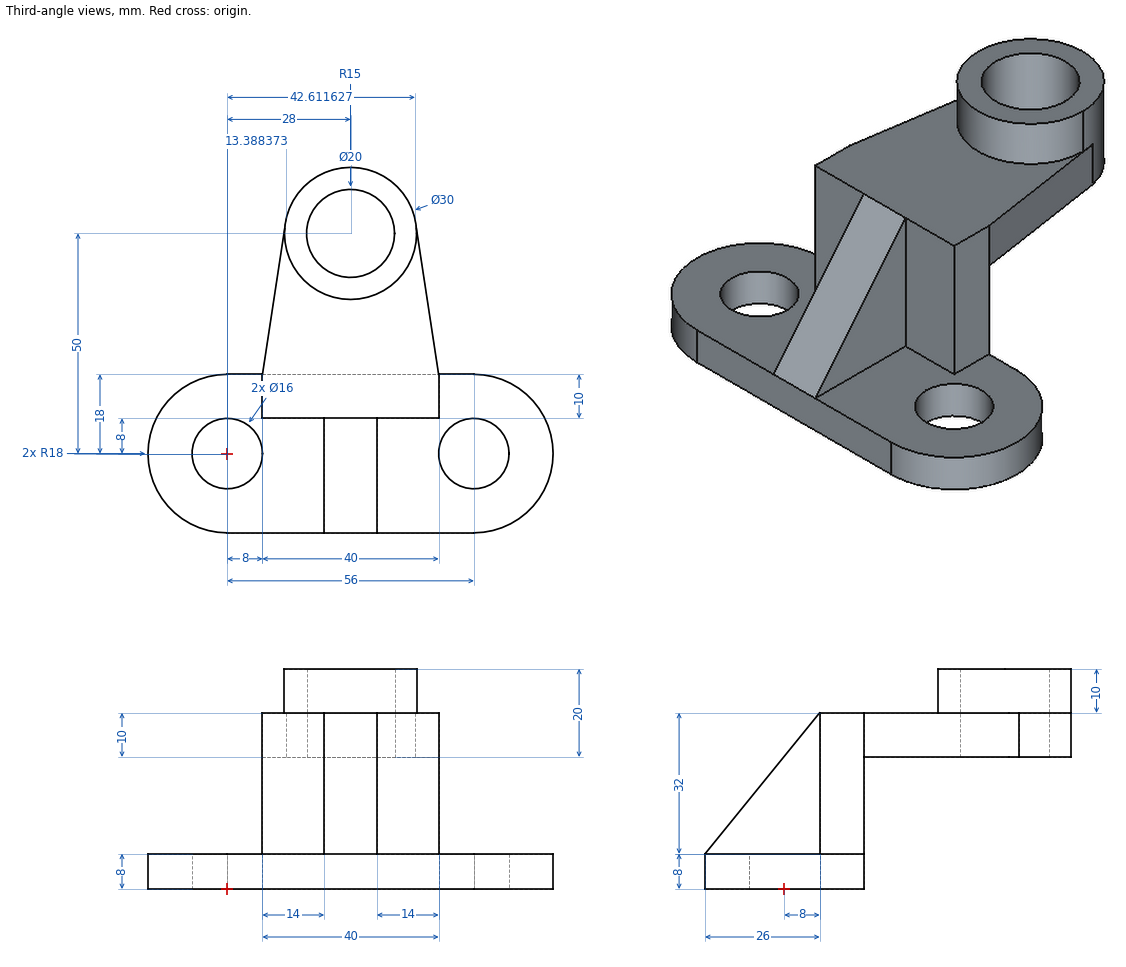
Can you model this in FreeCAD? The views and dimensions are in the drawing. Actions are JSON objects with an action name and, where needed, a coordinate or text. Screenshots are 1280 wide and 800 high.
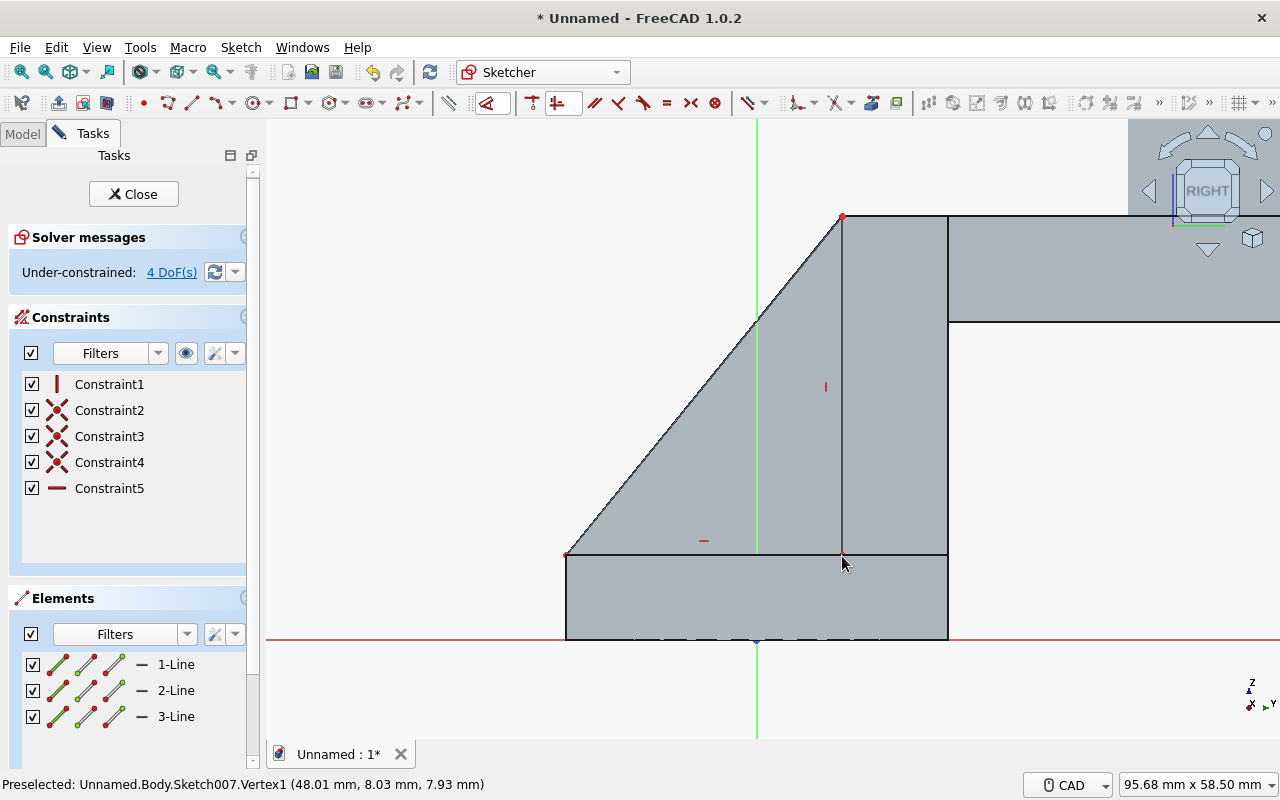
{"action": "left_click", "coordinate": [842, 454]}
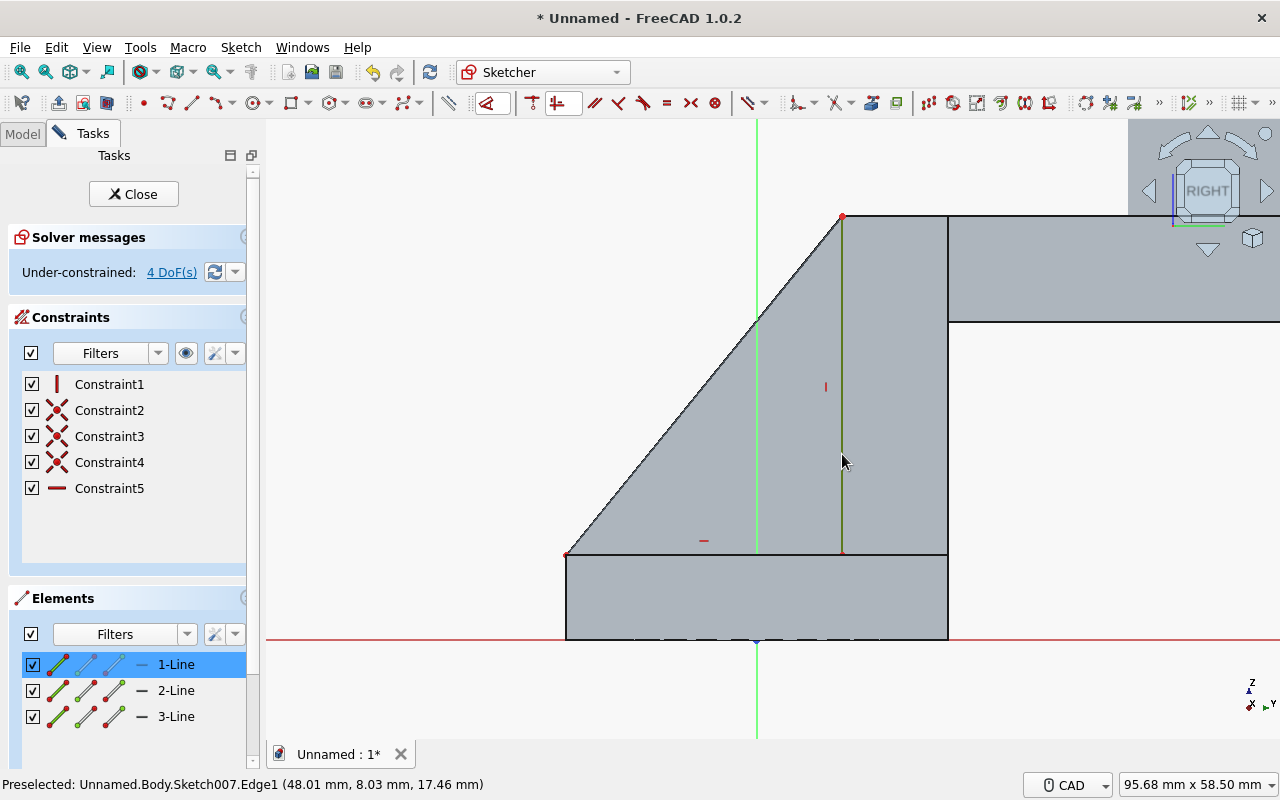
{"action": "key", "text": "i"}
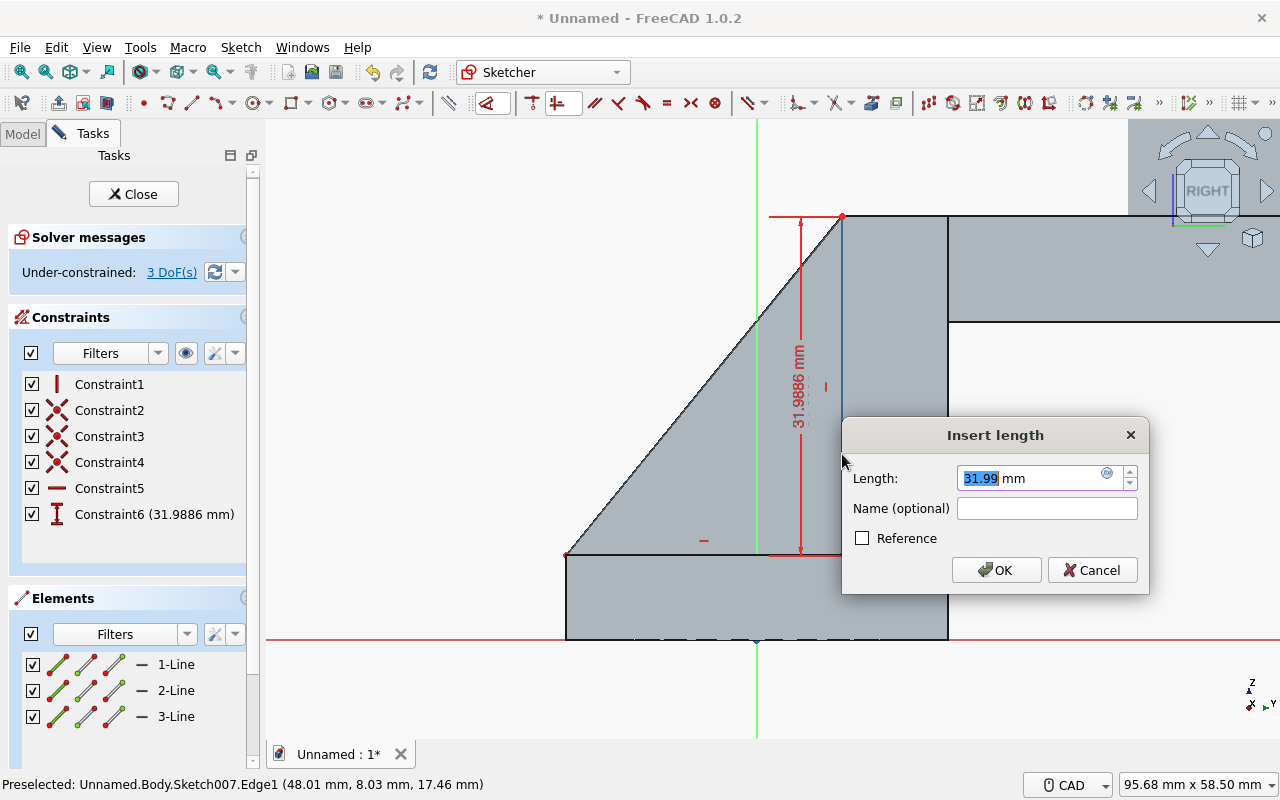
{"action": "type", "text": "32"}
{"action": "key", "text": "Return"}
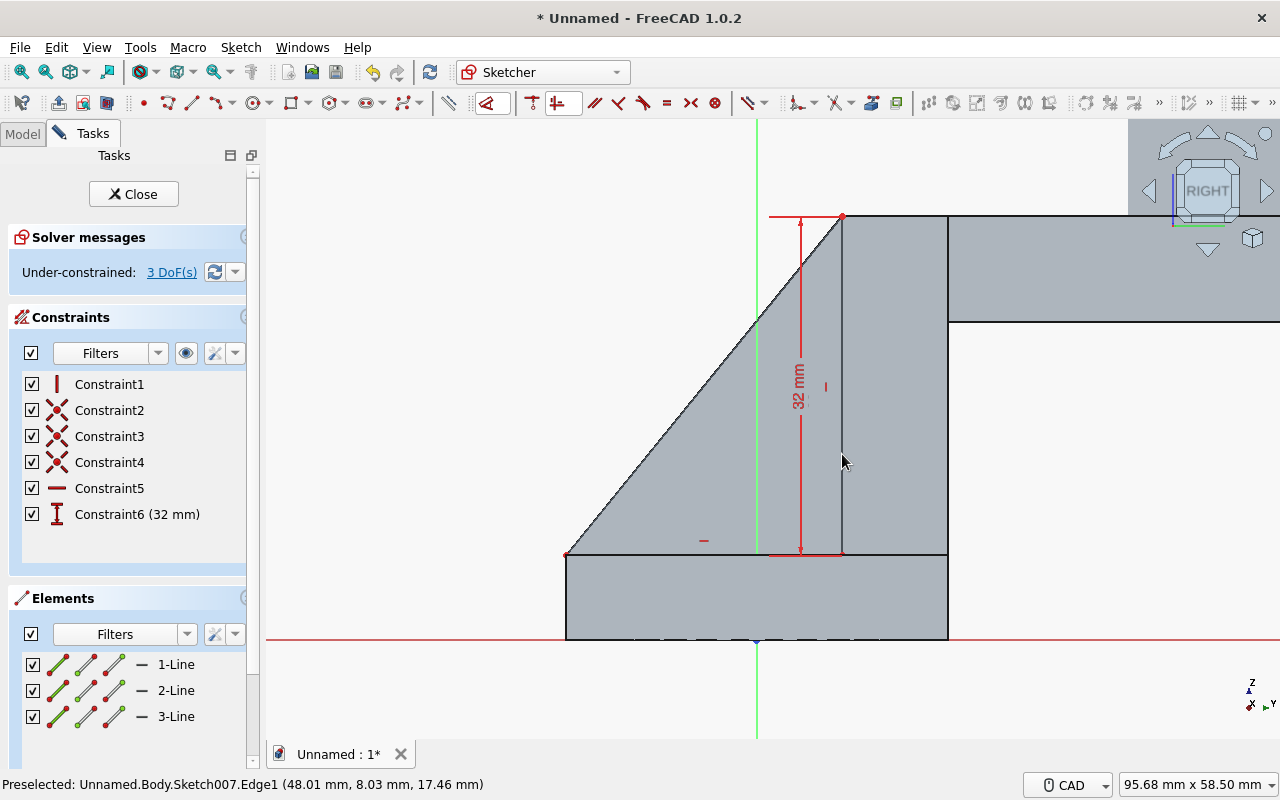
{"action": "left_click", "coordinate": [649, 556]}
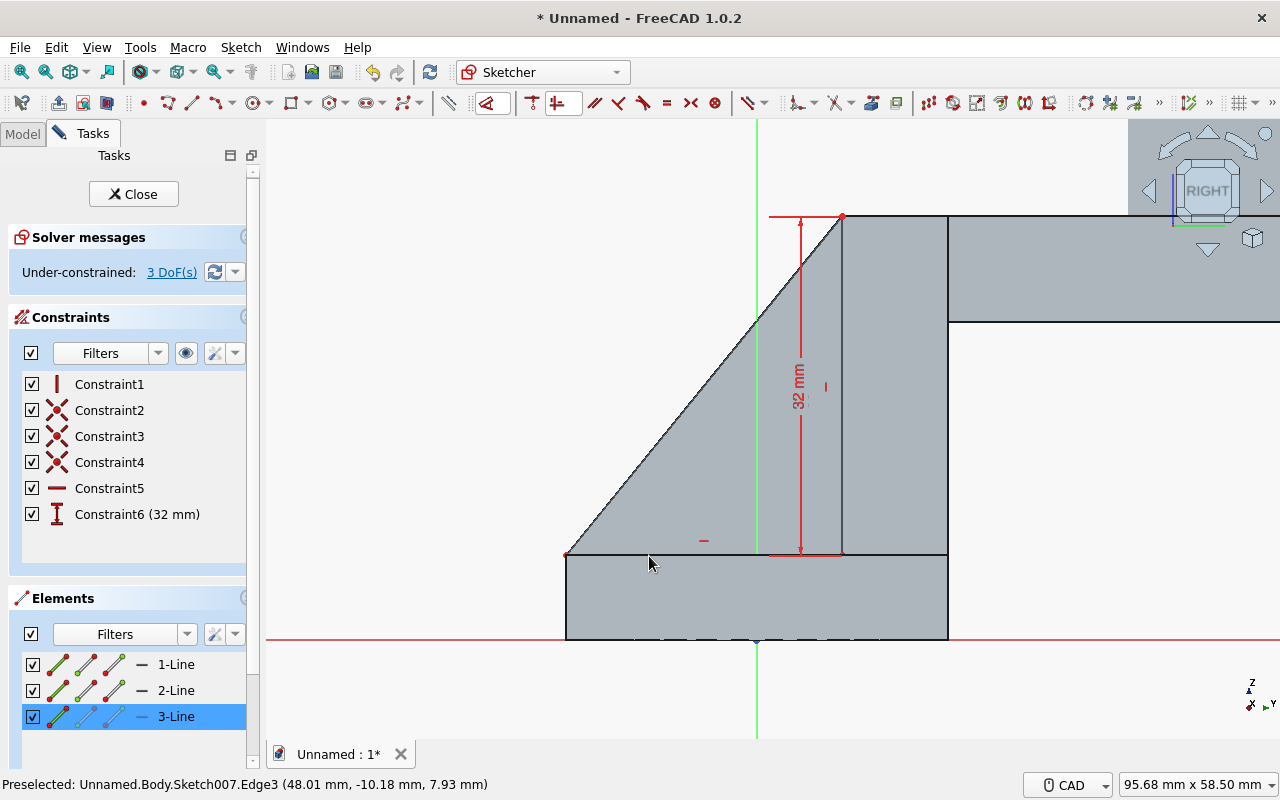
{"action": "left_click", "coordinate": [504, 104]}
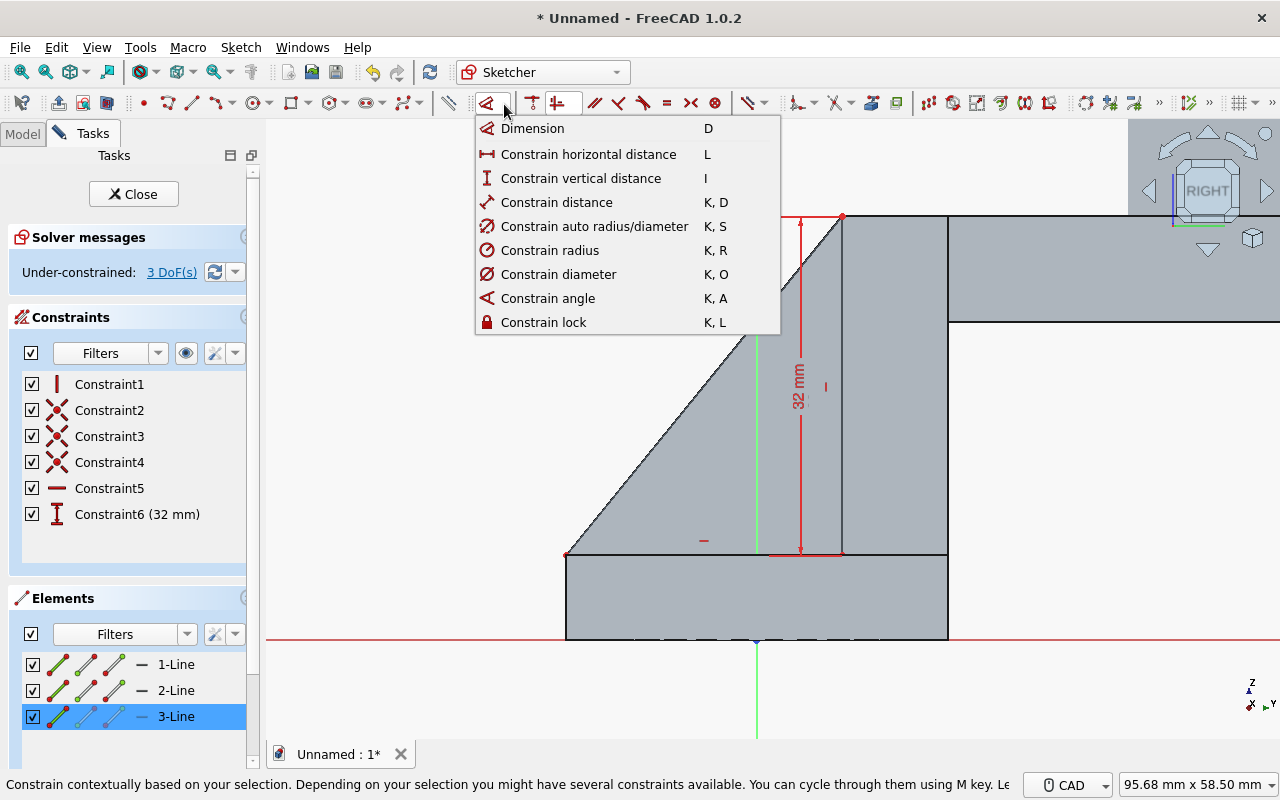
{"action": "left_click", "coordinate": [628, 154]}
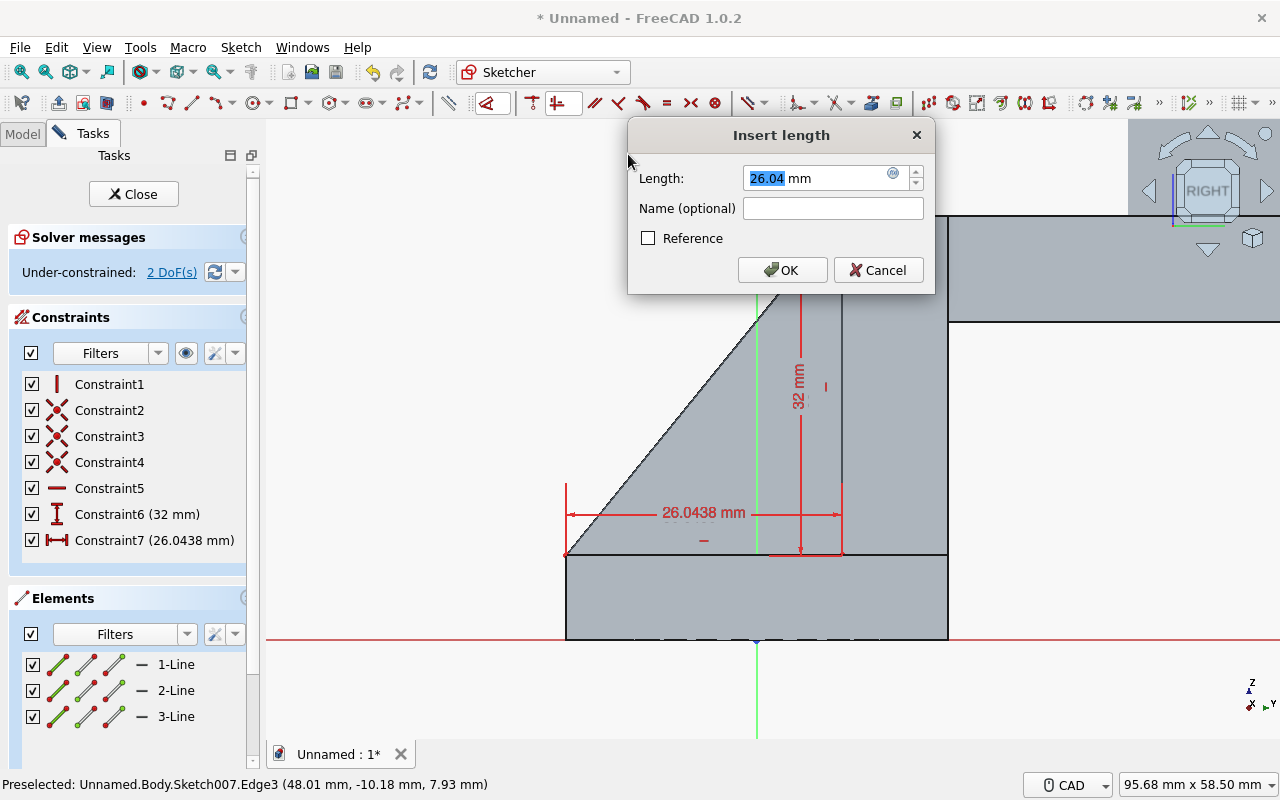
{"action": "type", "text": "26"}
{"action": "key", "text": "Return"}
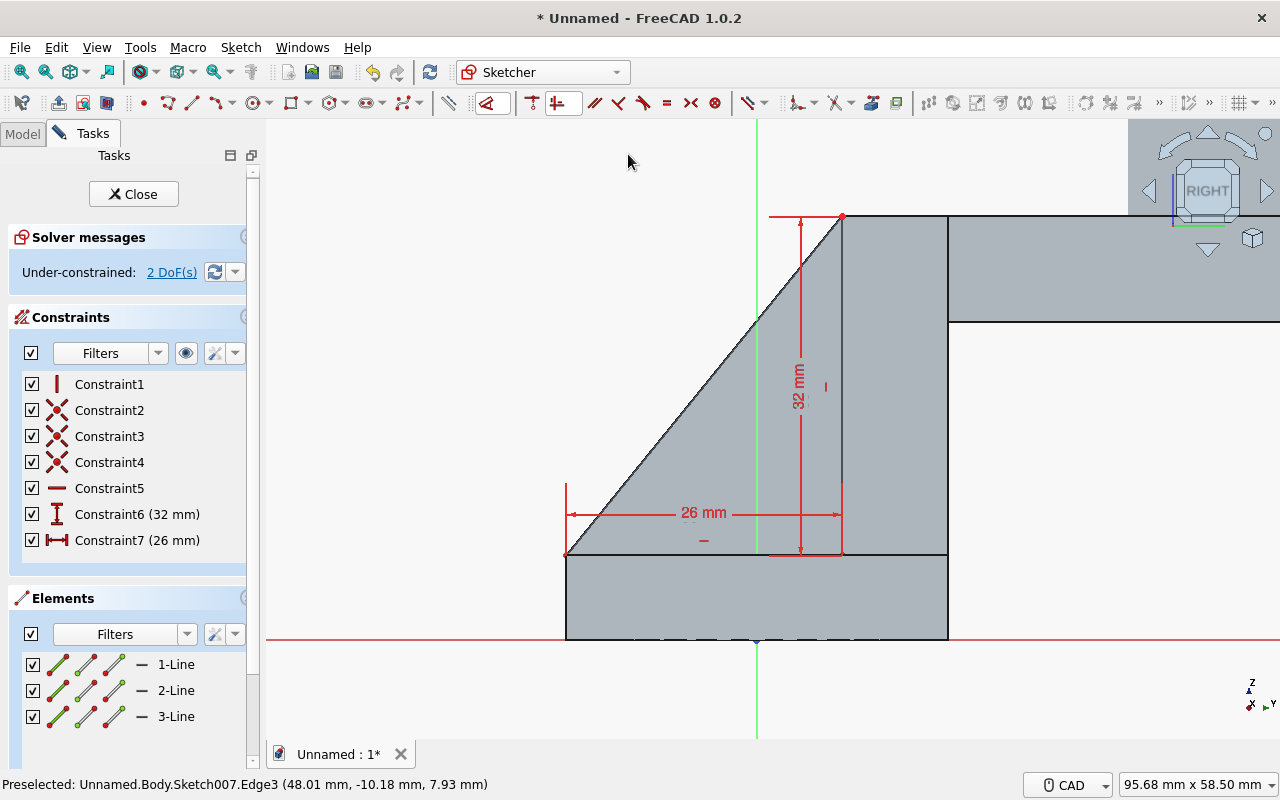
{"action": "left_click", "coordinate": [842, 556]}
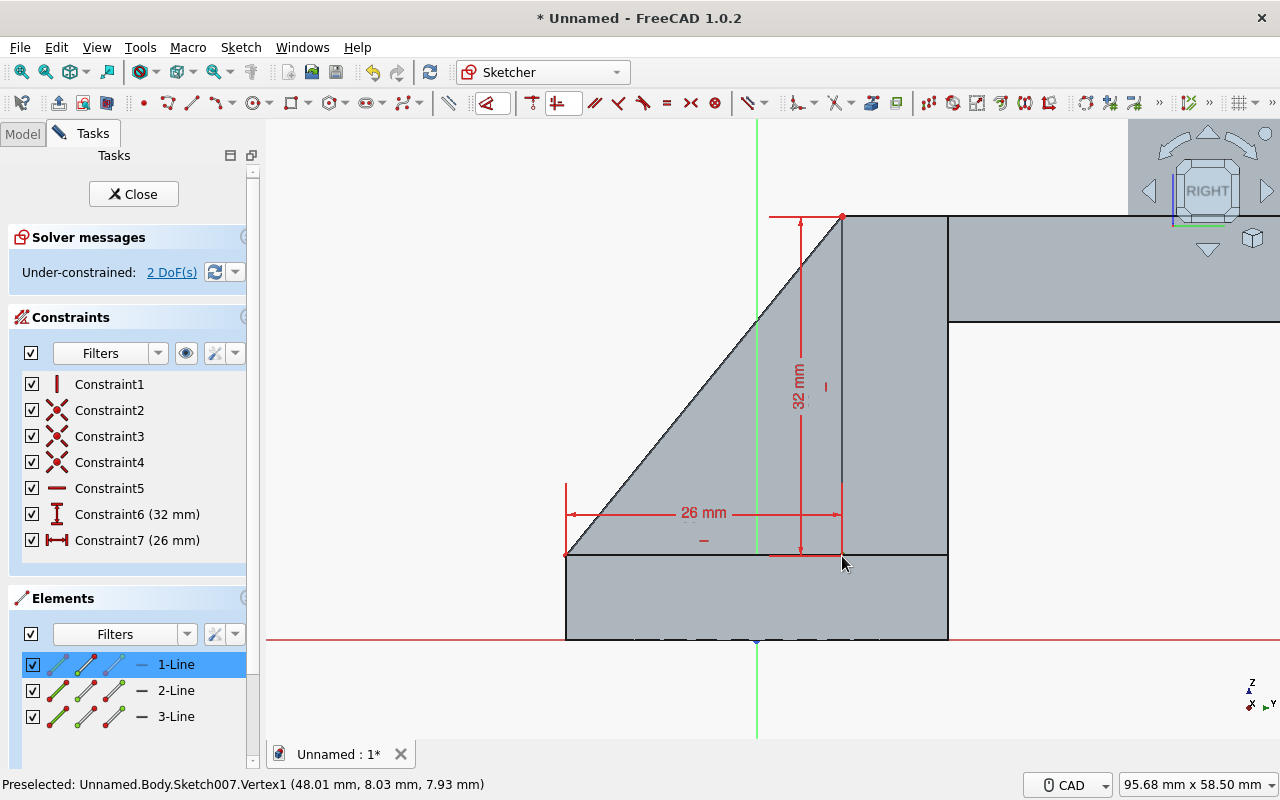
{"action": "key", "text": "l"}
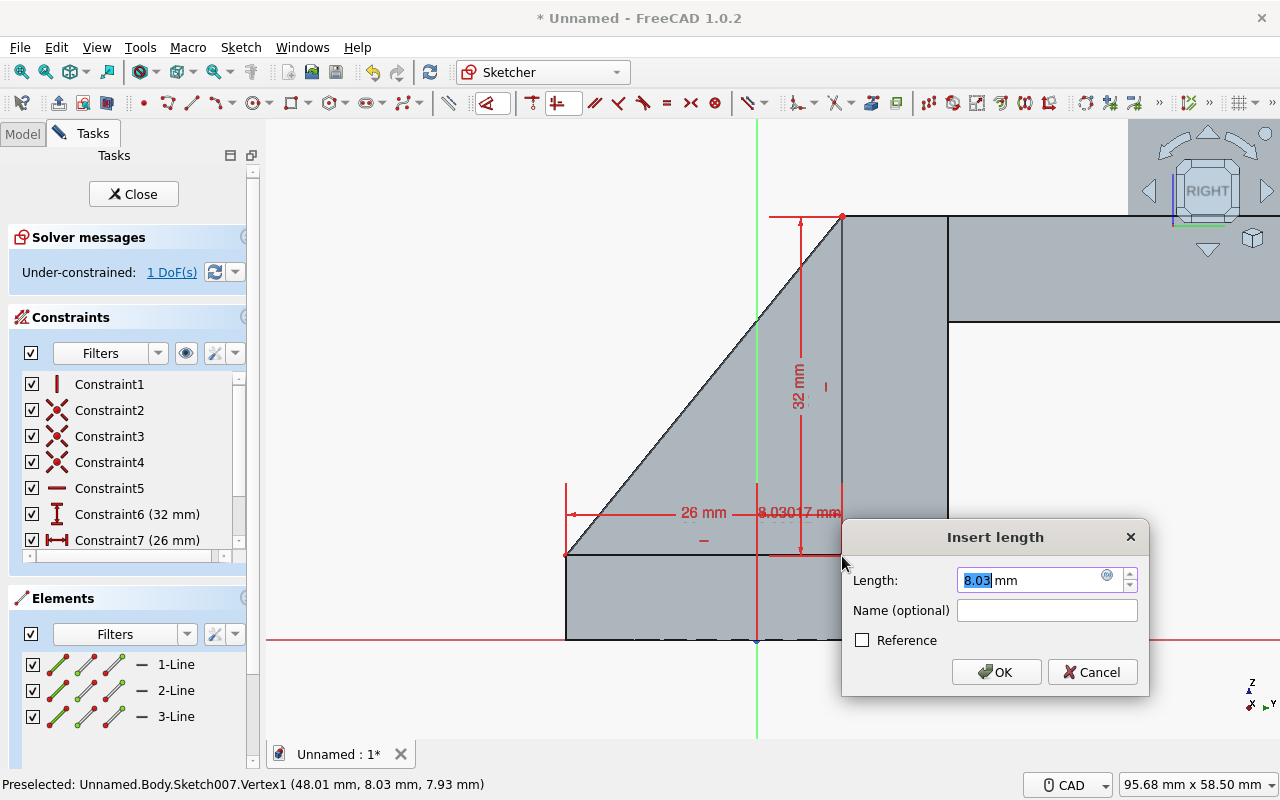
{"action": "type", "text": "8"}
{"action": "key", "text": "Return"}